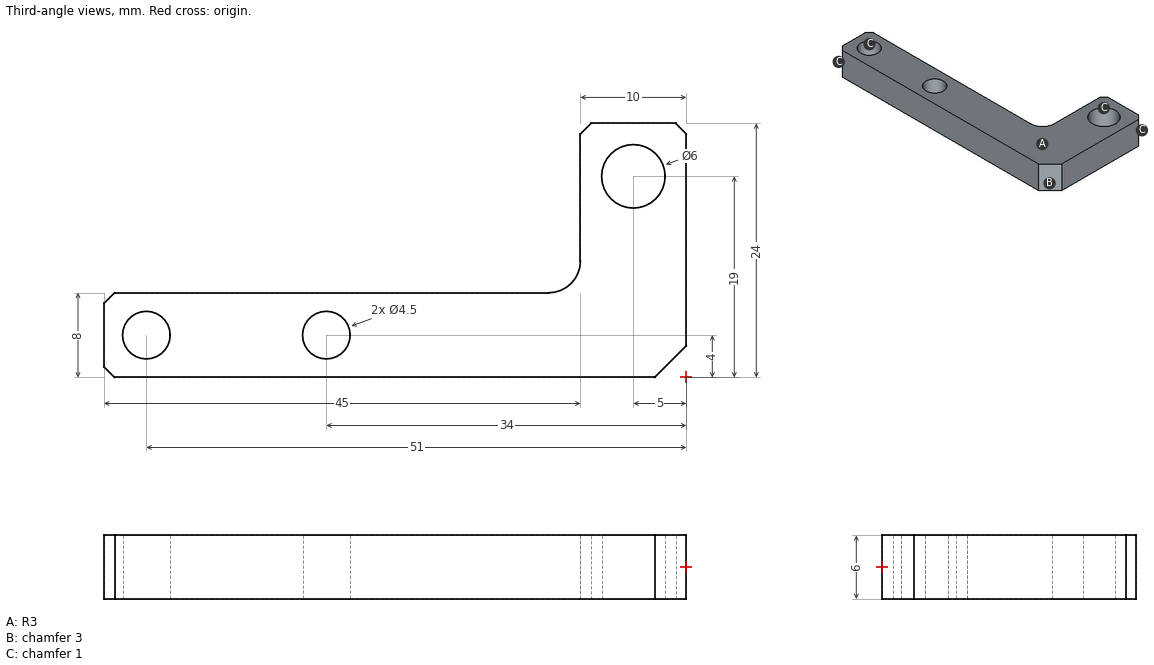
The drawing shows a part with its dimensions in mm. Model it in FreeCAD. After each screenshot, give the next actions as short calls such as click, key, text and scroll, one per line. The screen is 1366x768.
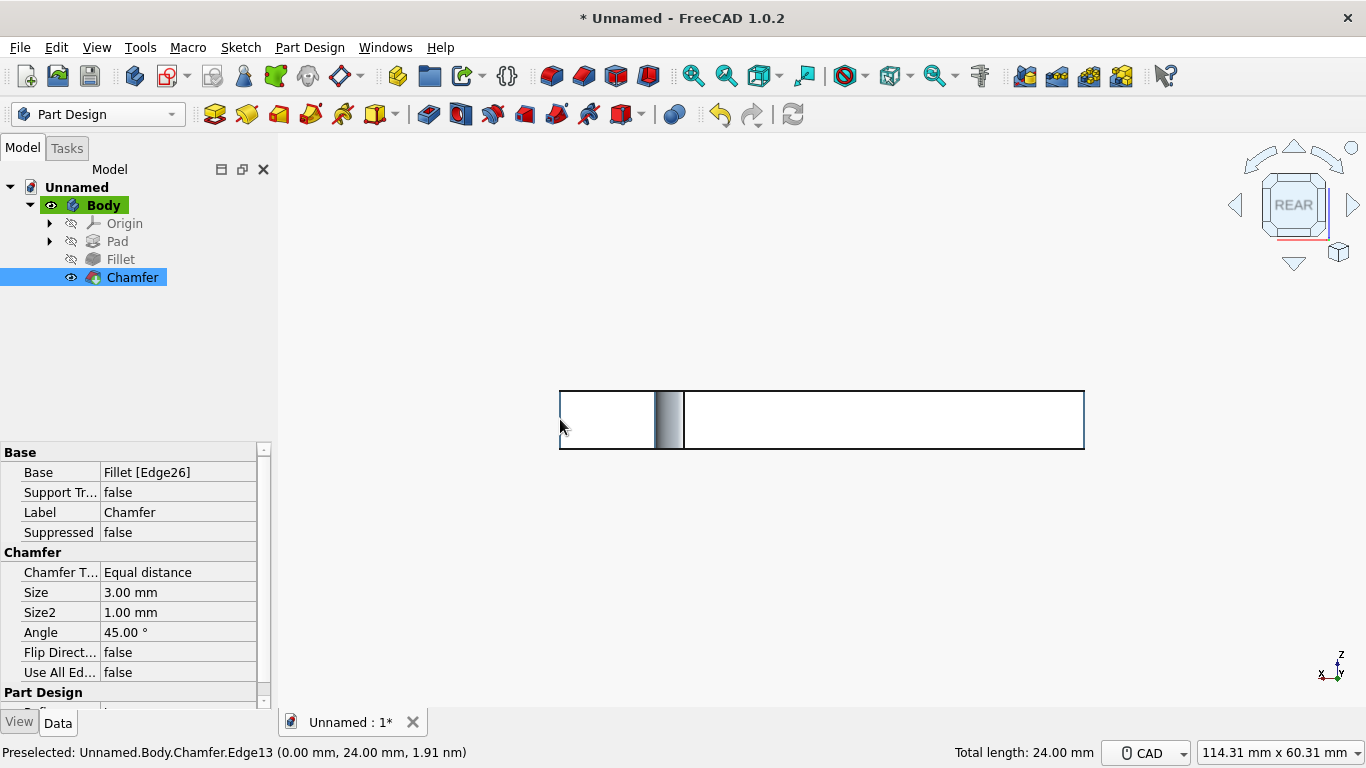
click(584, 76)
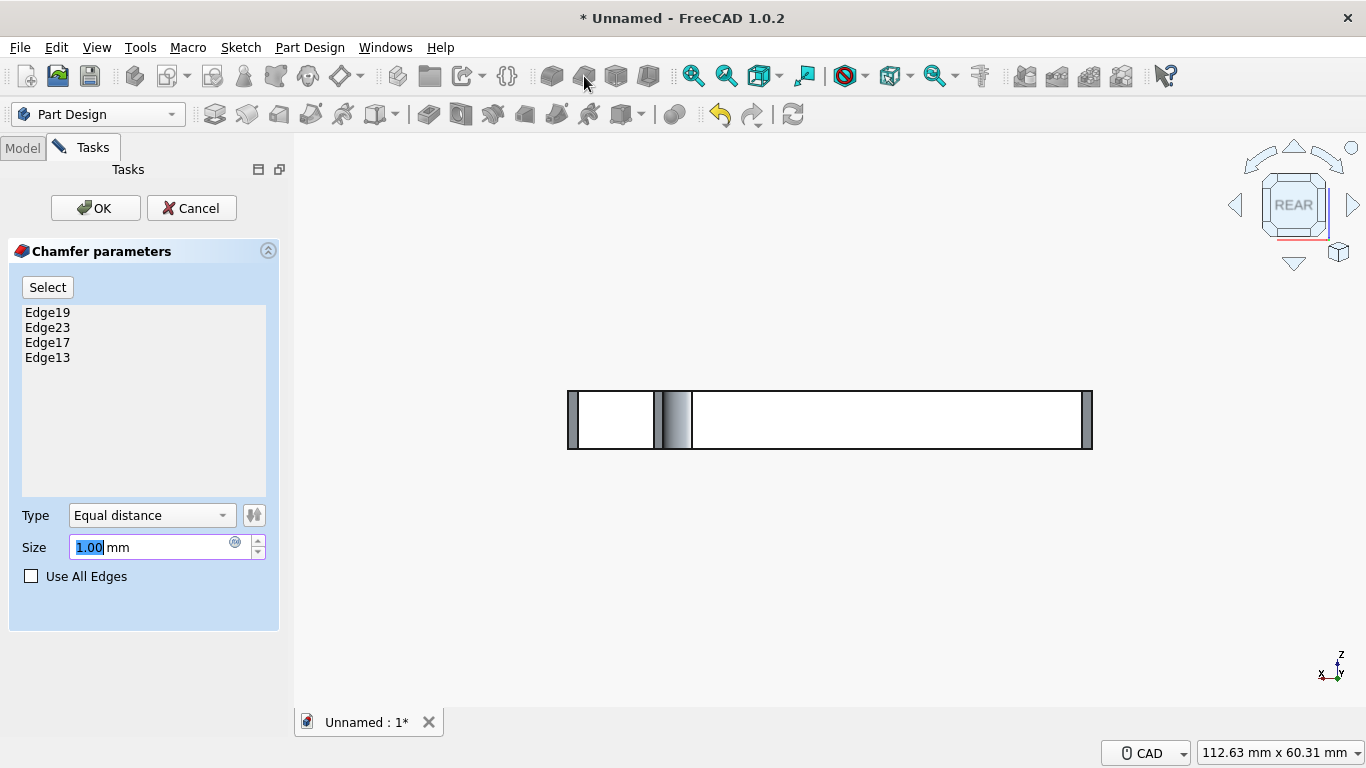
text(1)
key(Tab)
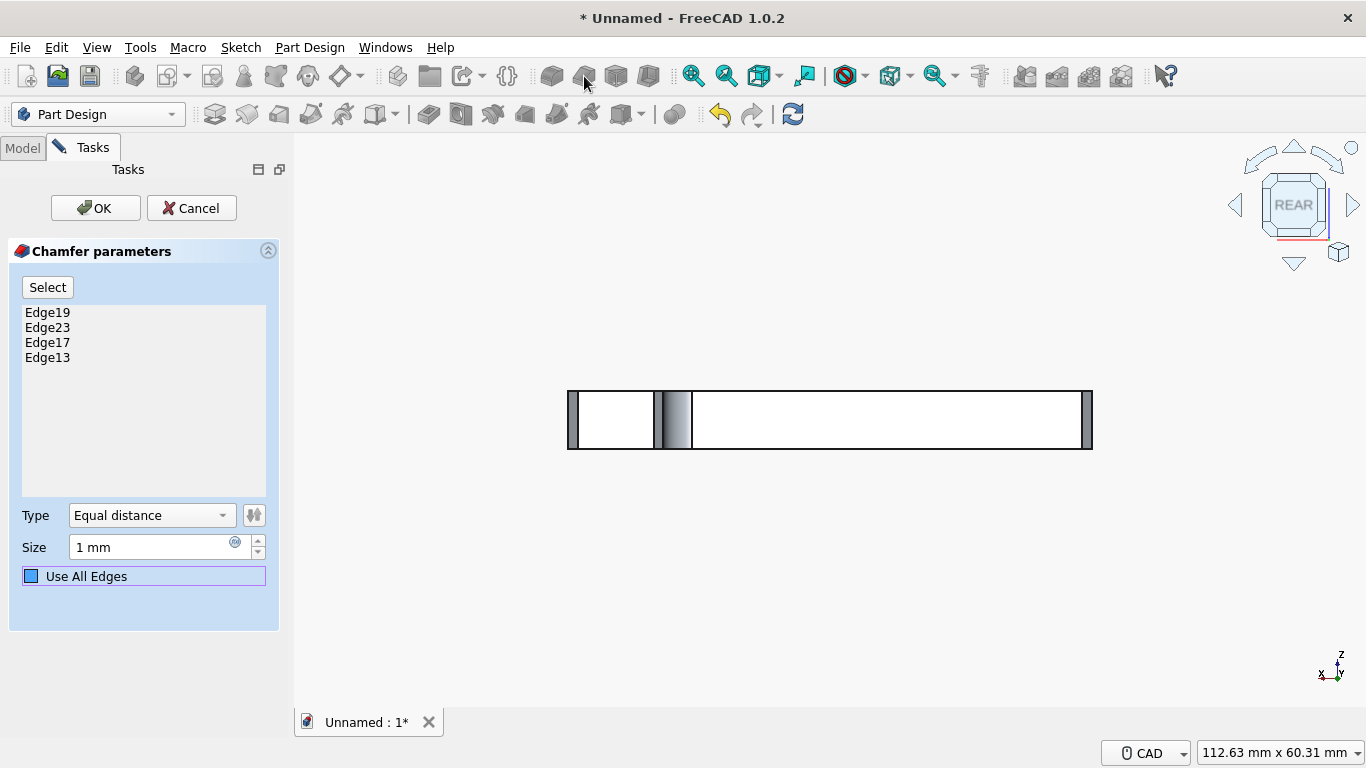
click(96, 208)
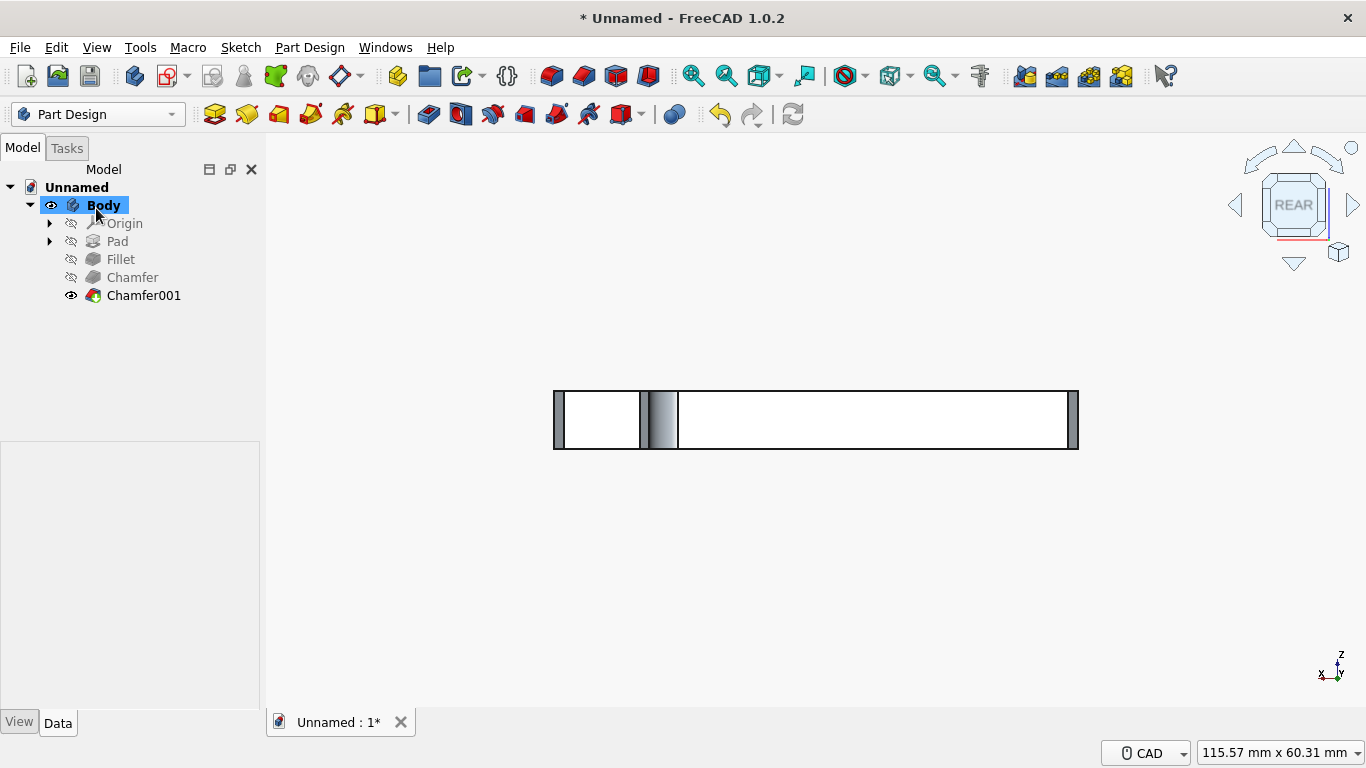
key(0)